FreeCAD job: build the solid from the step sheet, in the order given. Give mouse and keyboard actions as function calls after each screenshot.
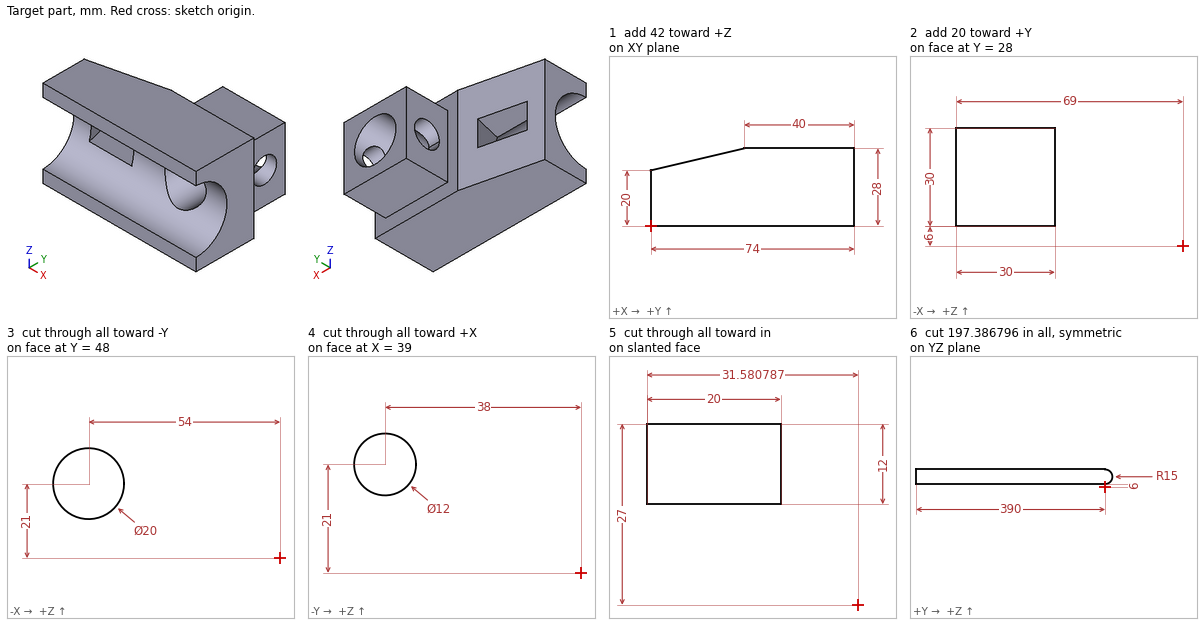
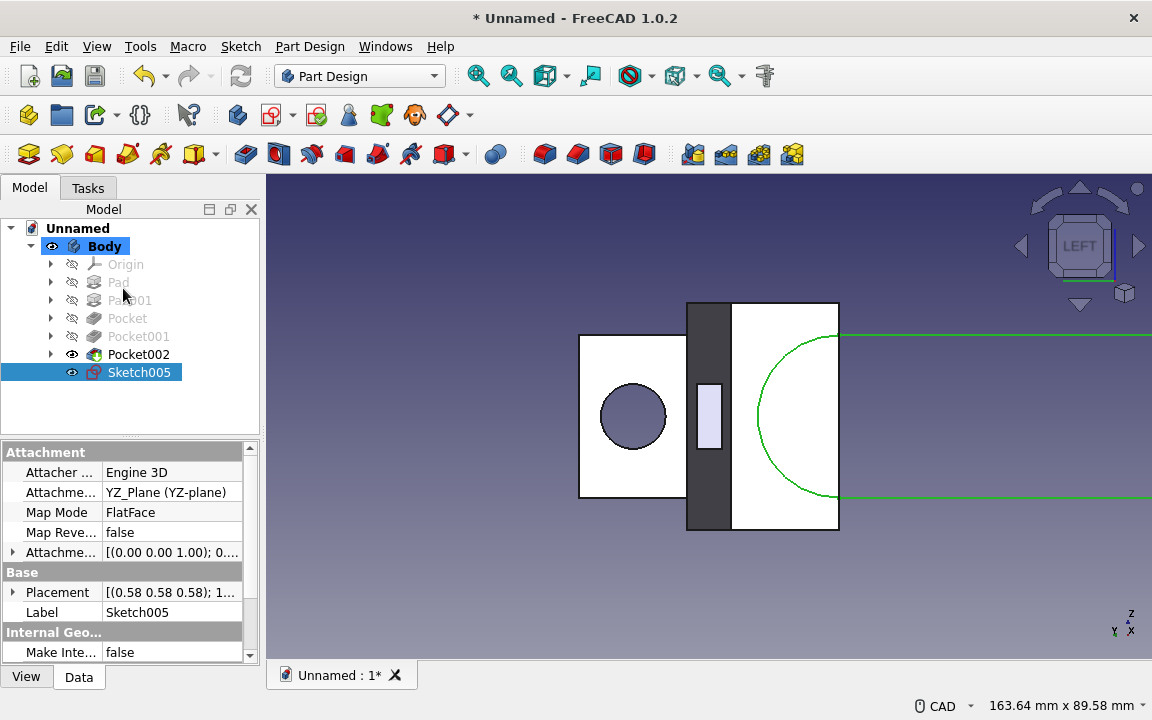
click(246, 154)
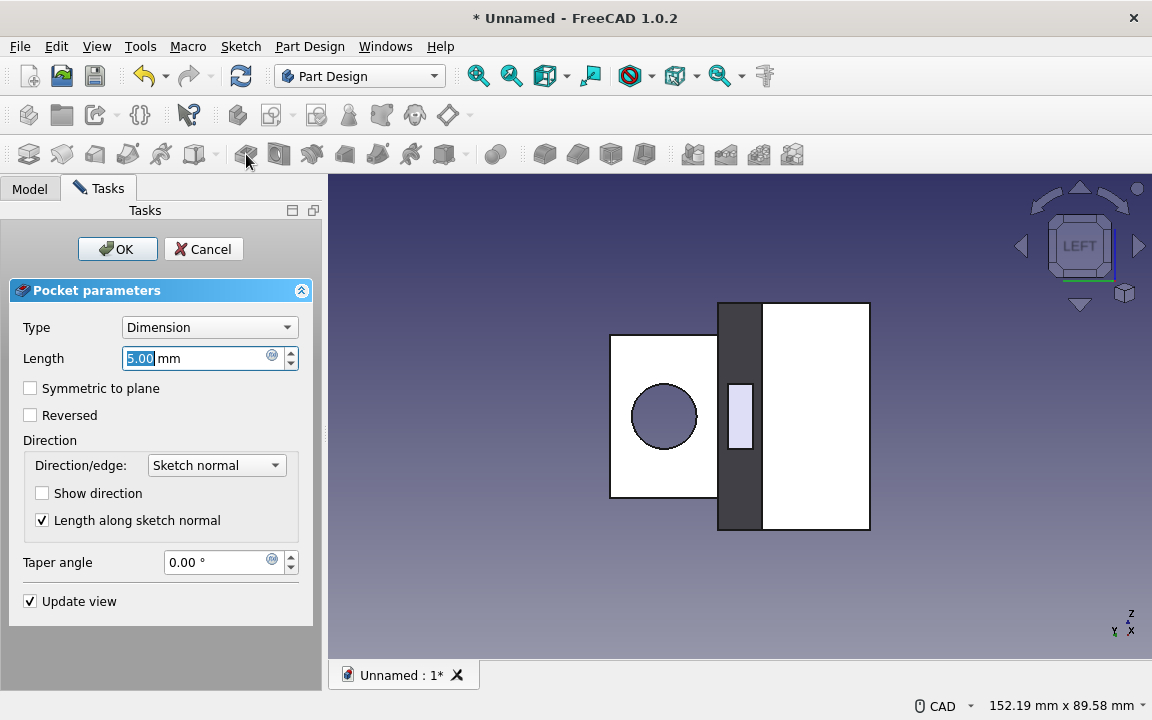
text(197.386796)
key(Tab)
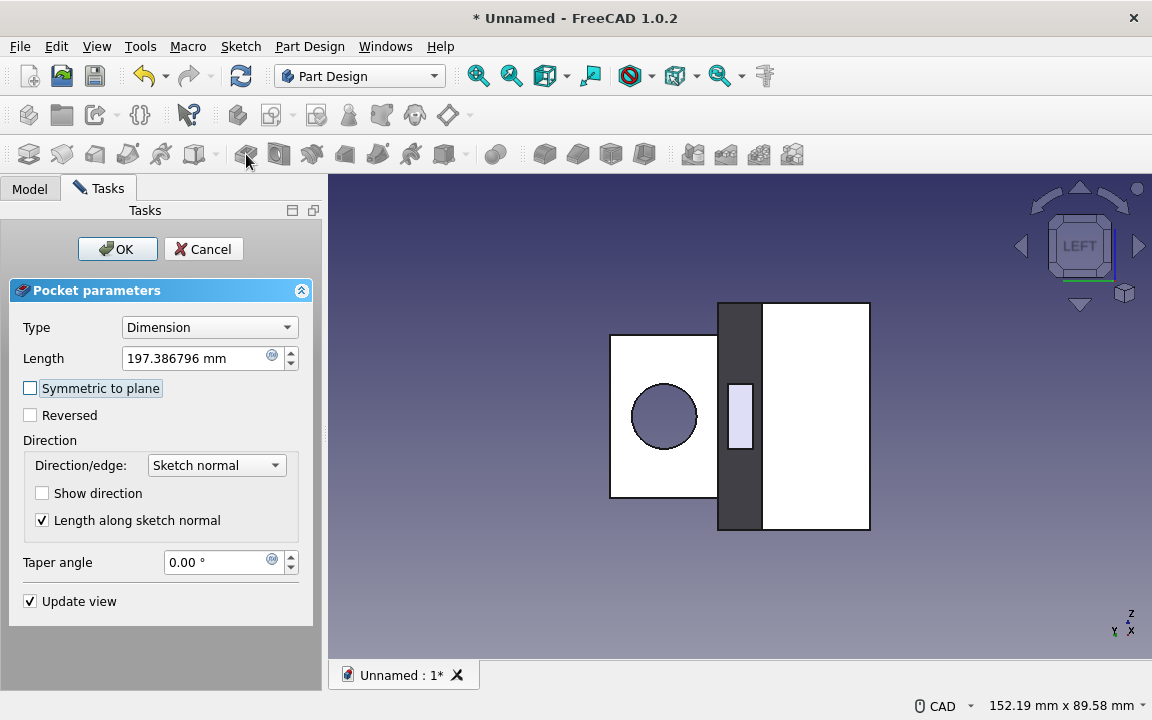
click(31, 388)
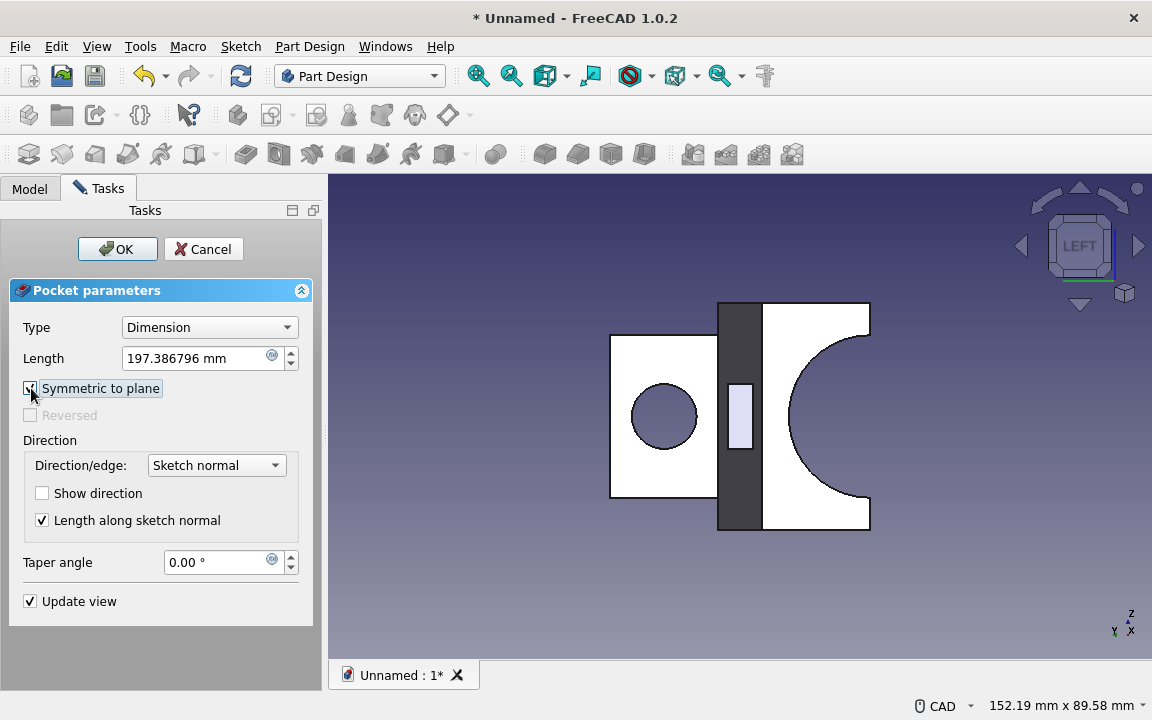
click(118, 249)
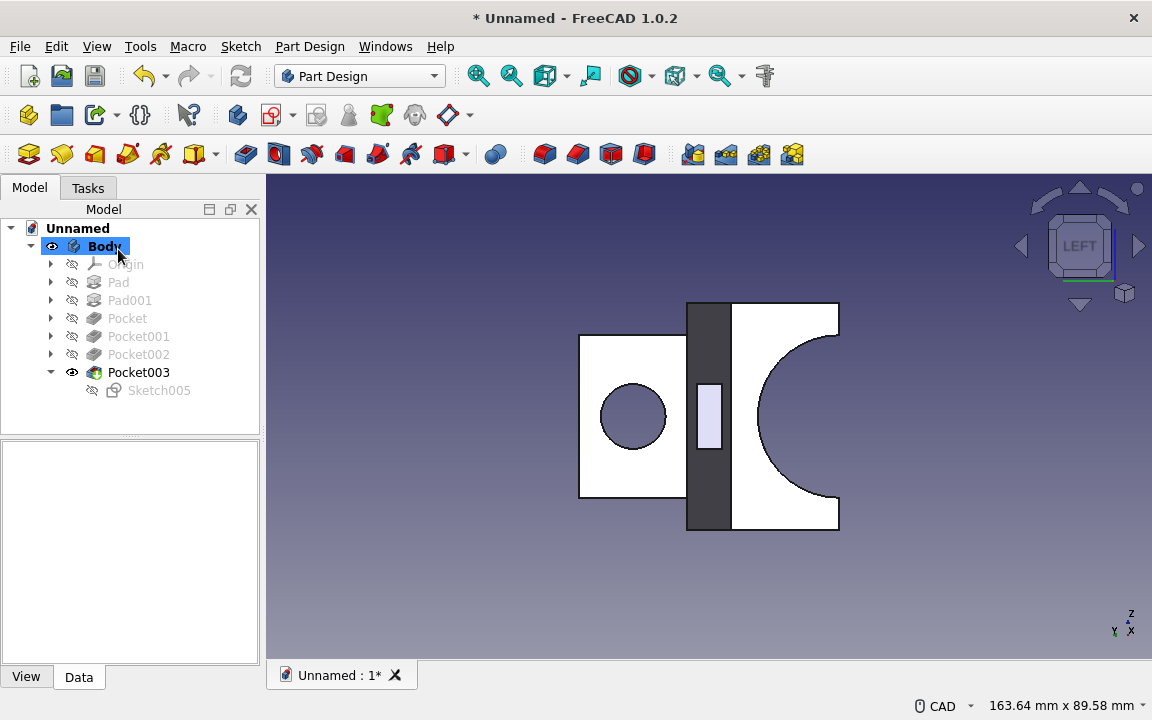
key(0)